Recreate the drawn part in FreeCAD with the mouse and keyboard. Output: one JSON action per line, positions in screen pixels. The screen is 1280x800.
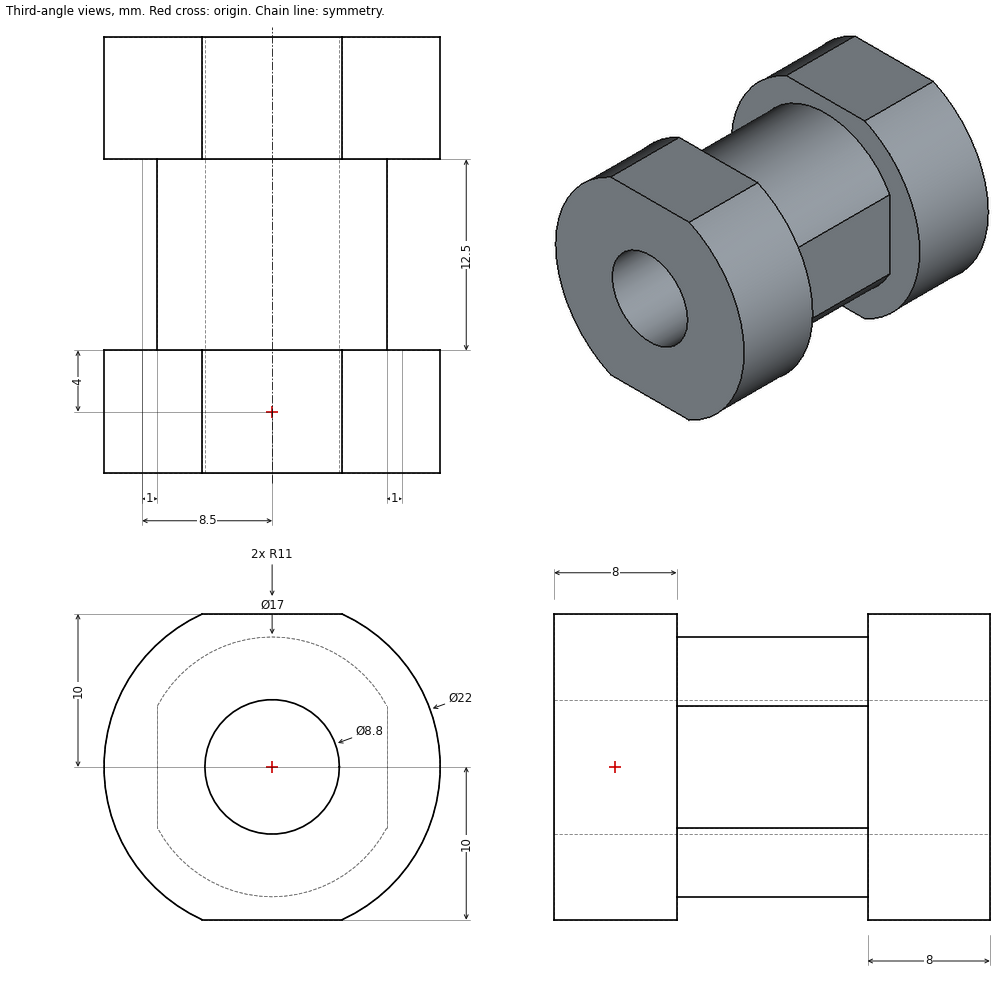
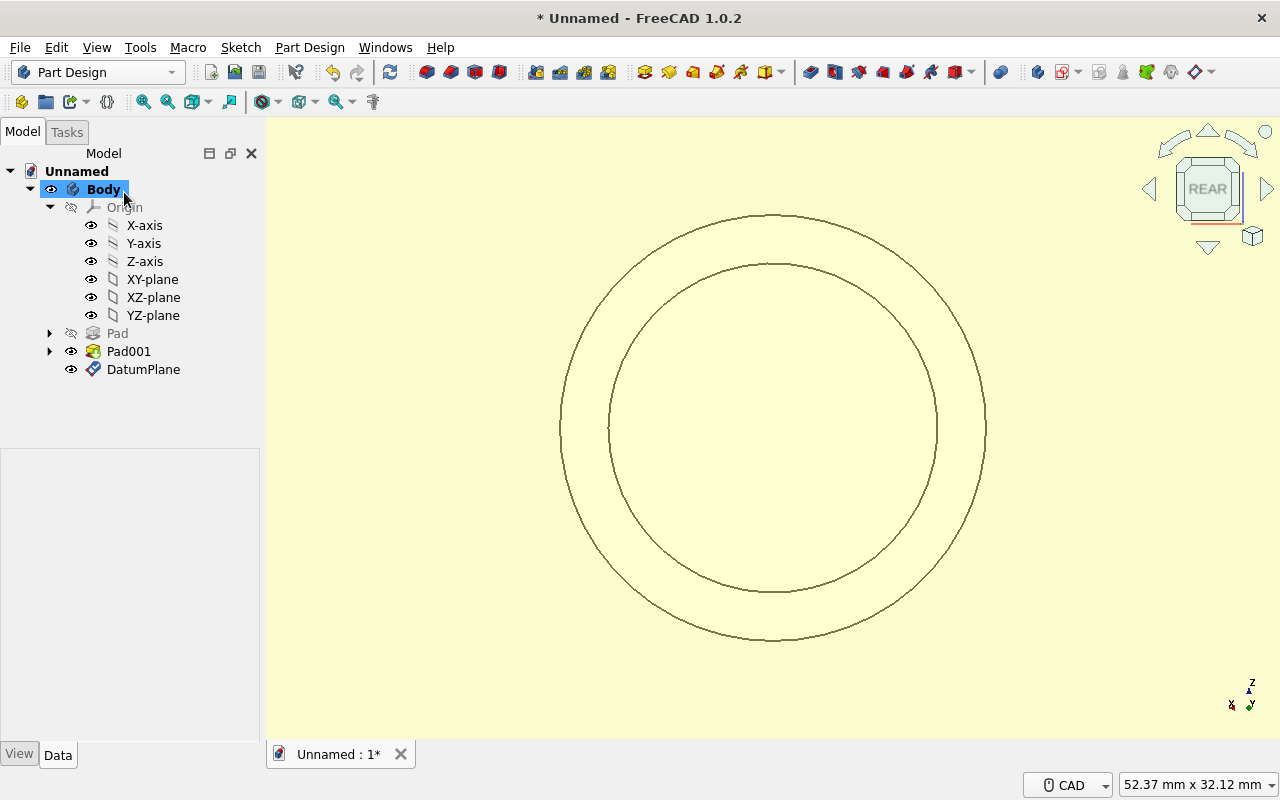
{"action": "left_click", "coordinate": [116, 369]}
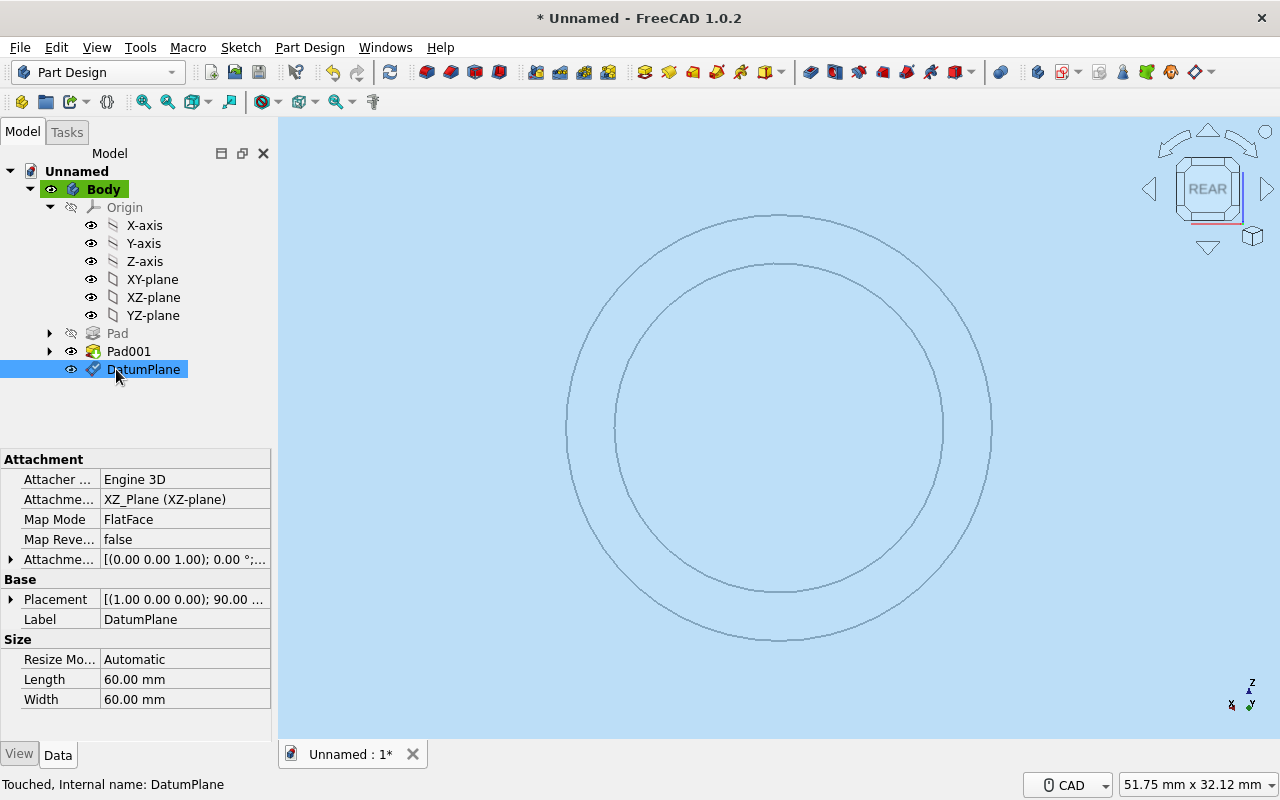
{"action": "left_click", "coordinate": [1062, 72]}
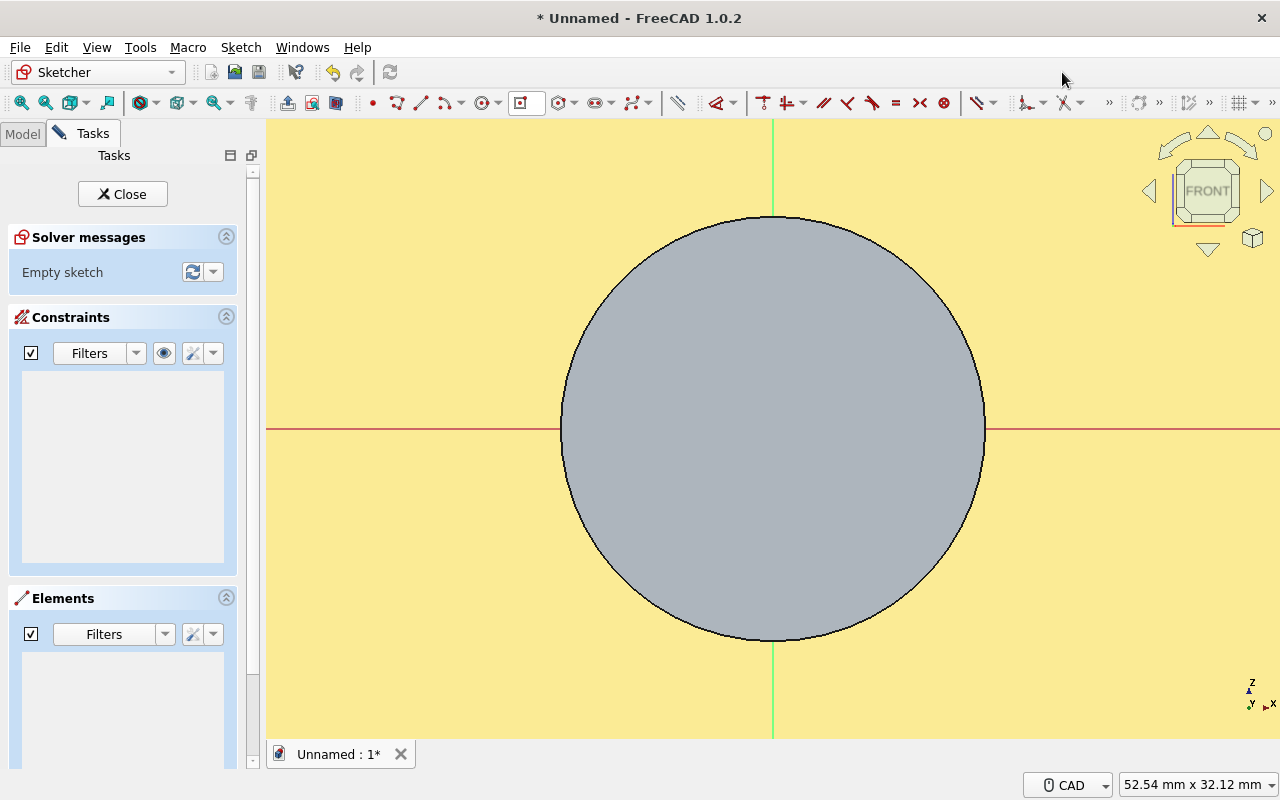
{"action": "key", "text": "q s"}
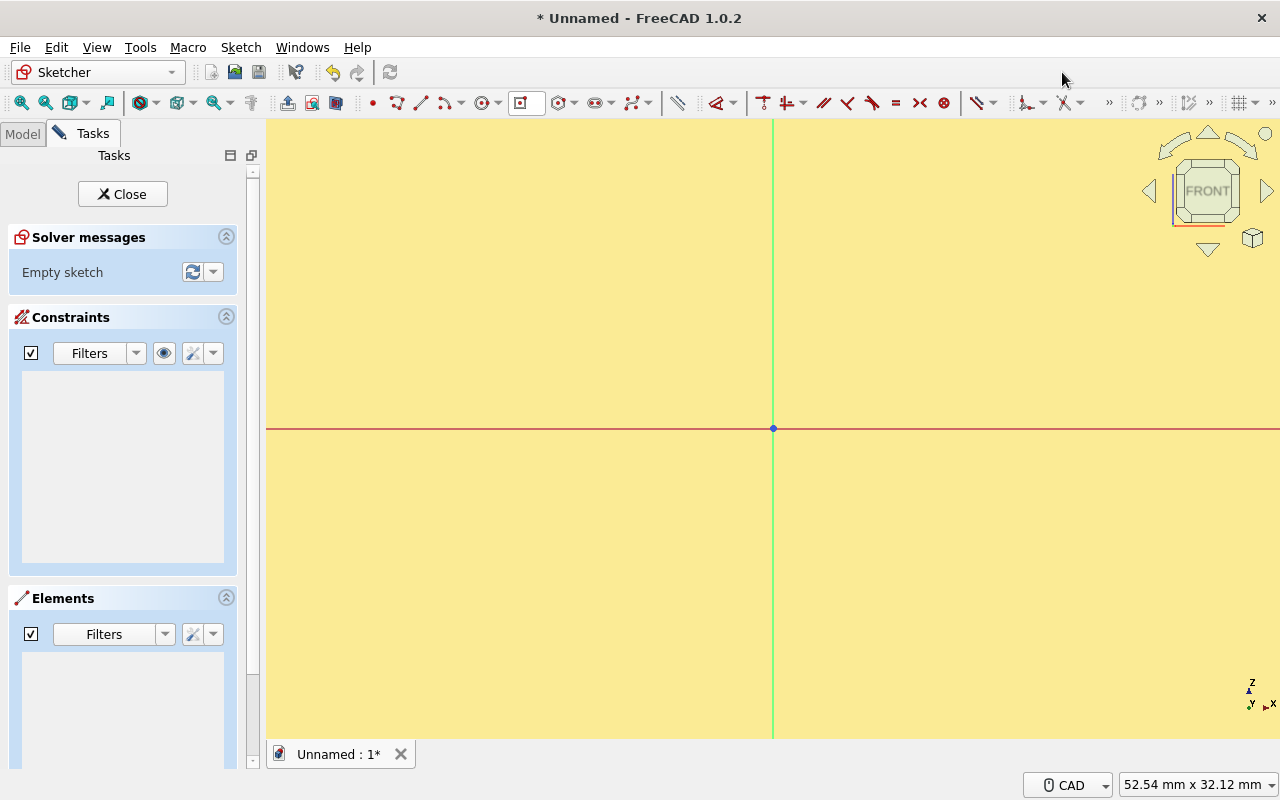
{"action": "left_click", "coordinate": [482, 104]}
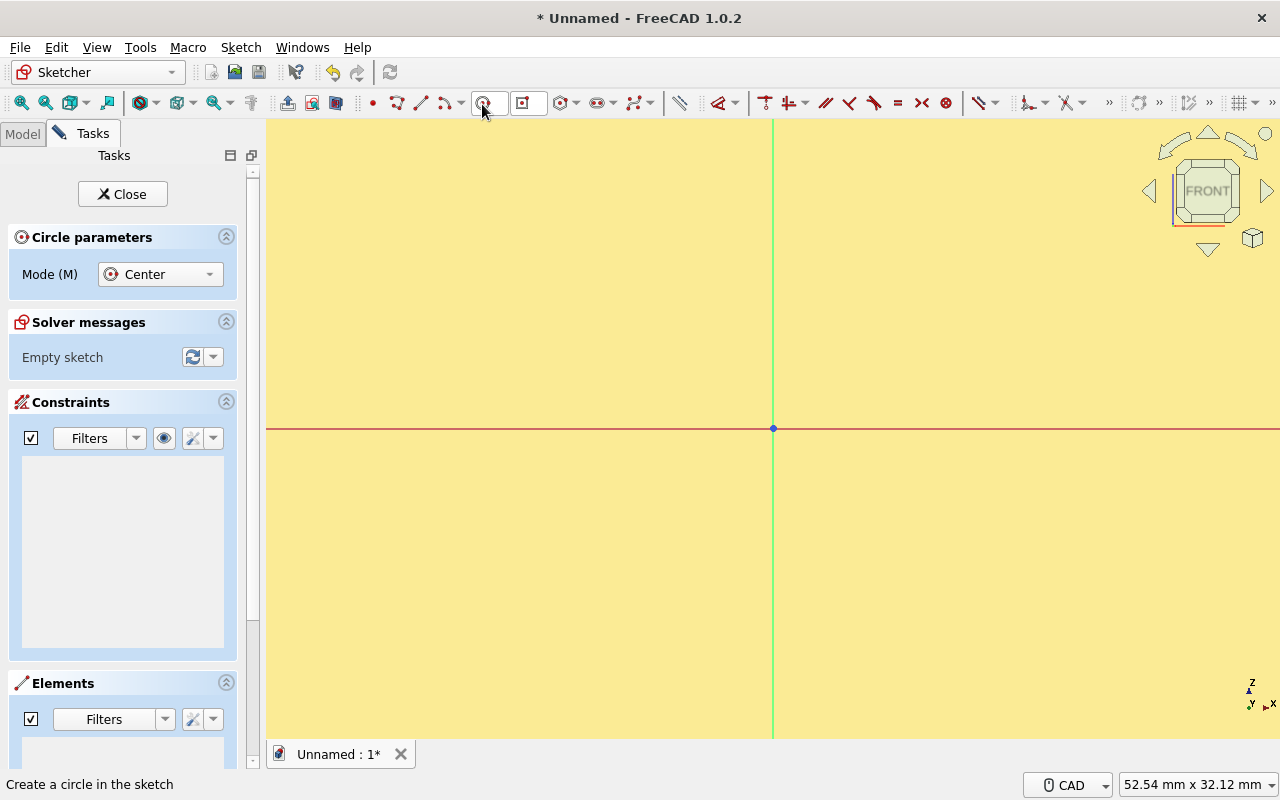
{"action": "left_click", "coordinate": [773, 429]}
{"action": "mouse_move", "coordinate": [923, 279]}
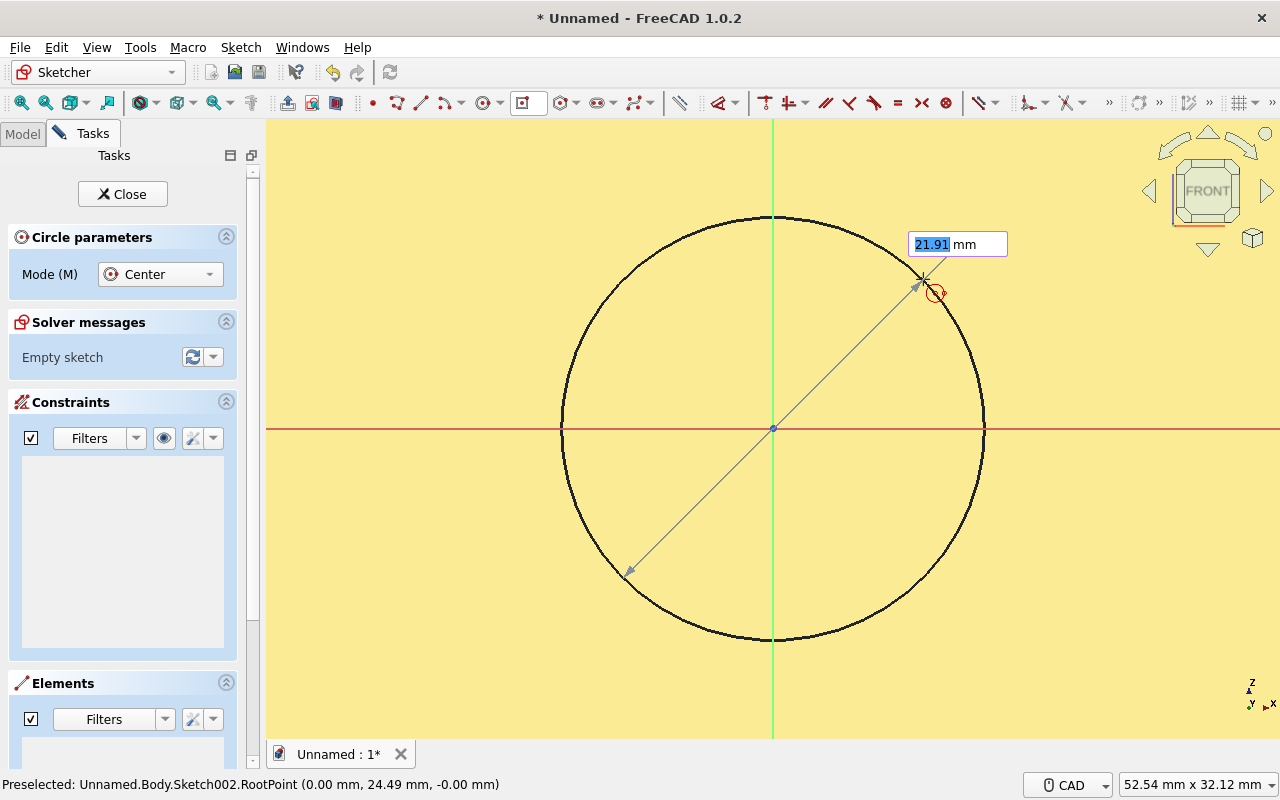
{"action": "type", "text": "22"}
{"action": "key", "text": "Return"}
{"action": "key", "text": "Escape"}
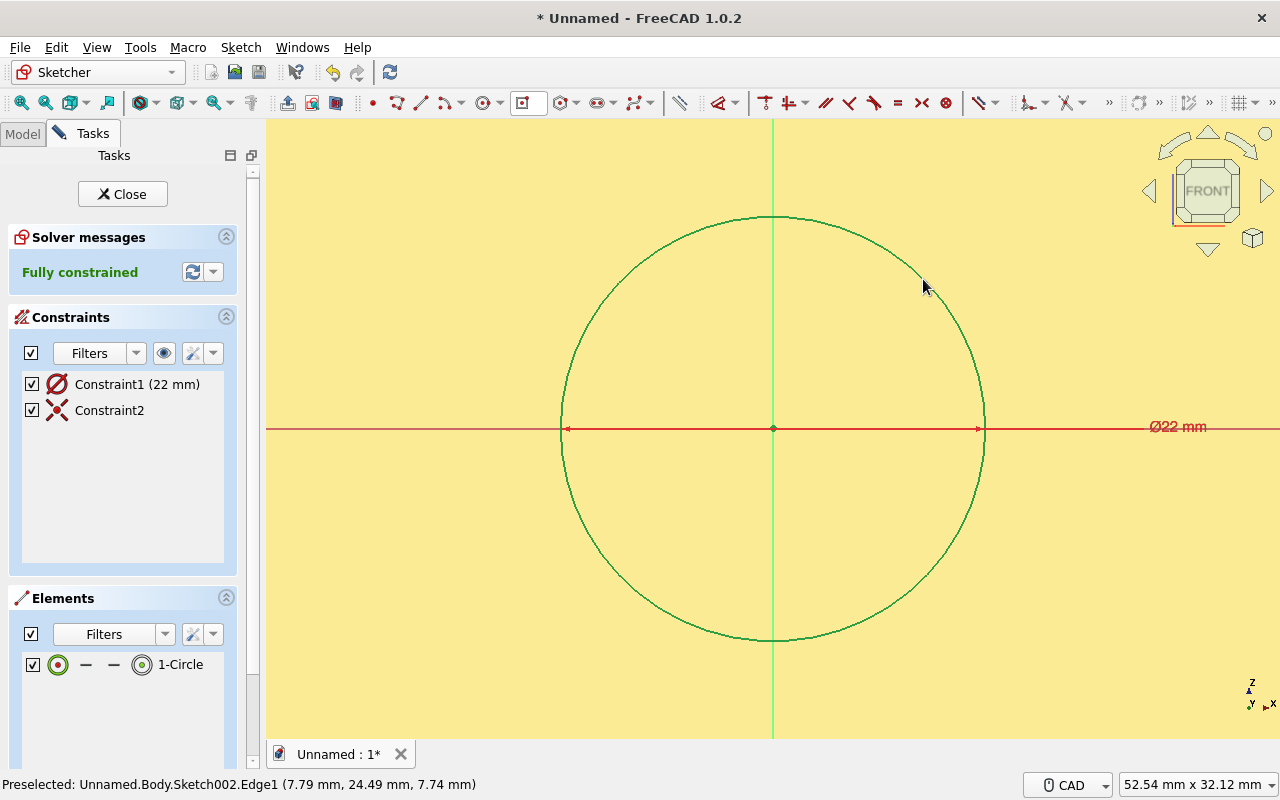
{"action": "left_click", "coordinate": [123, 194]}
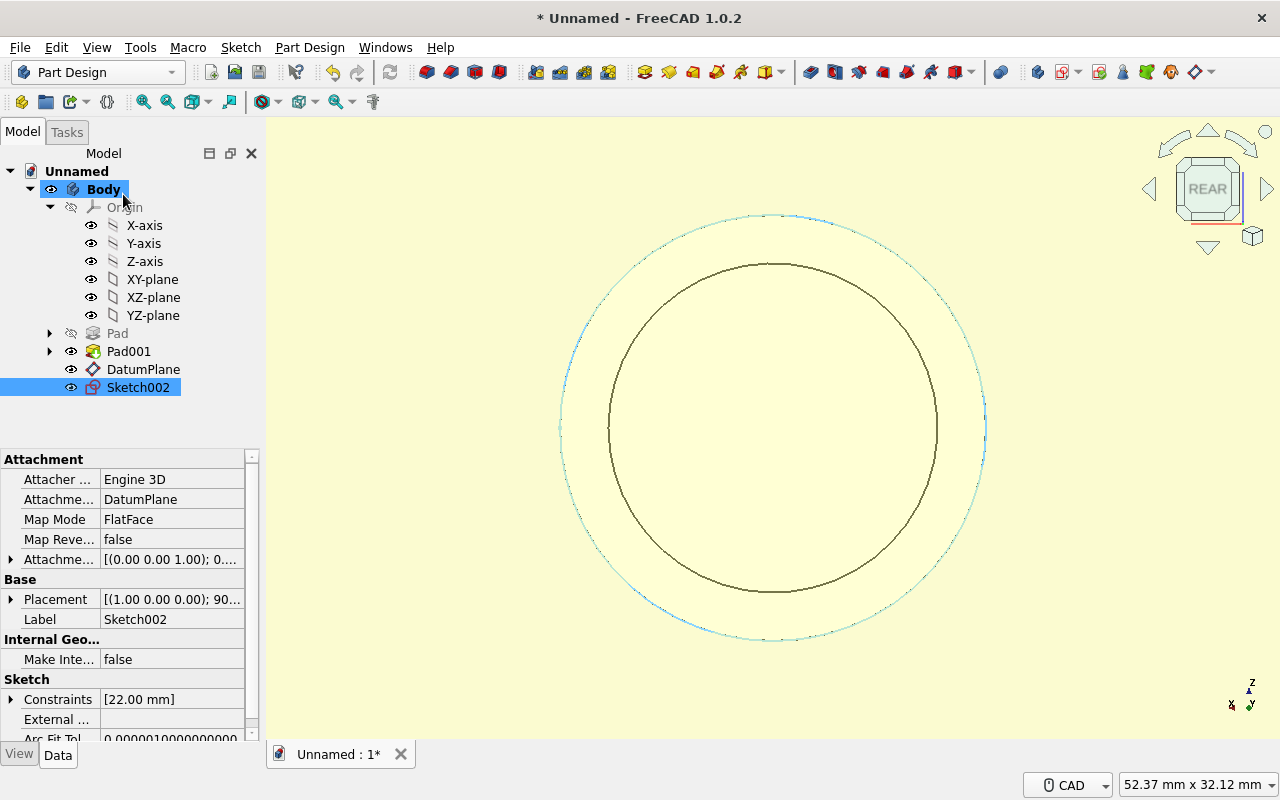
{"action": "left_click", "coordinate": [646, 72]}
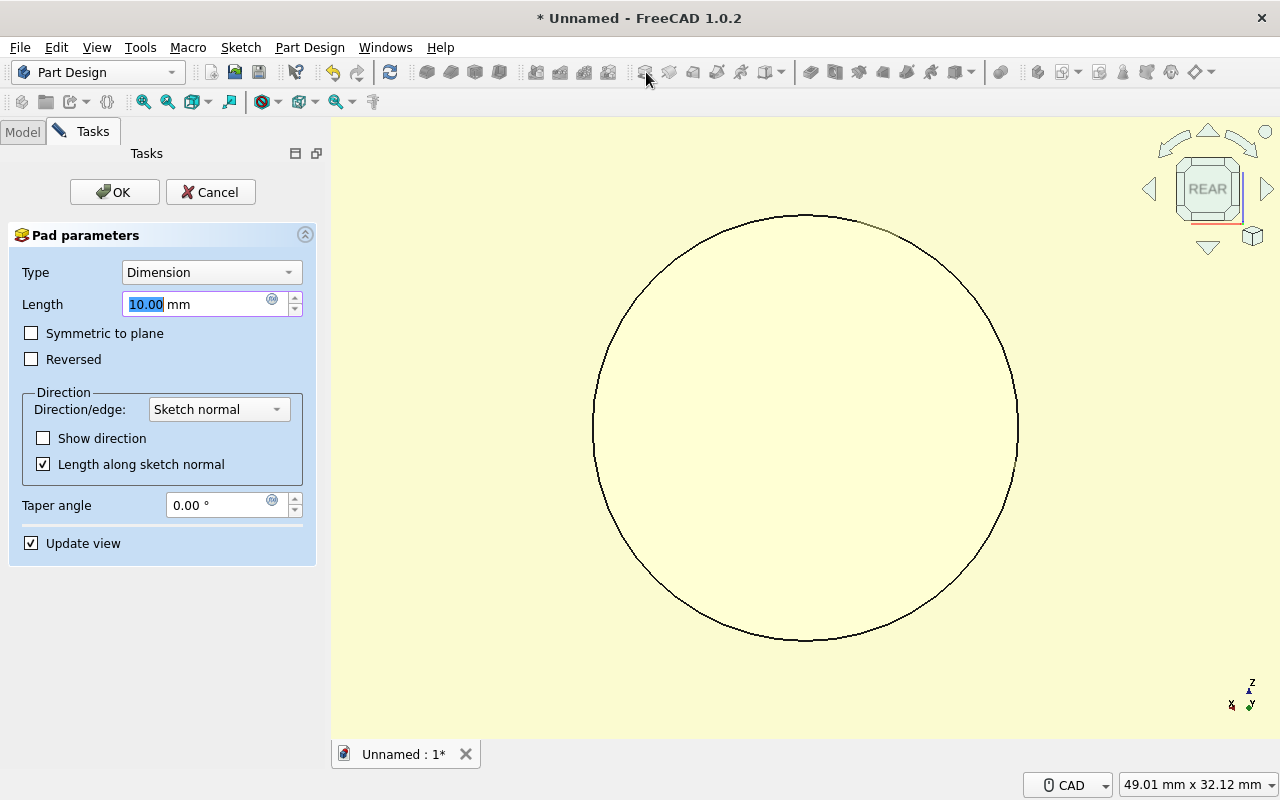
{"action": "type", "text": "8"}
{"action": "key", "text": "Tab"}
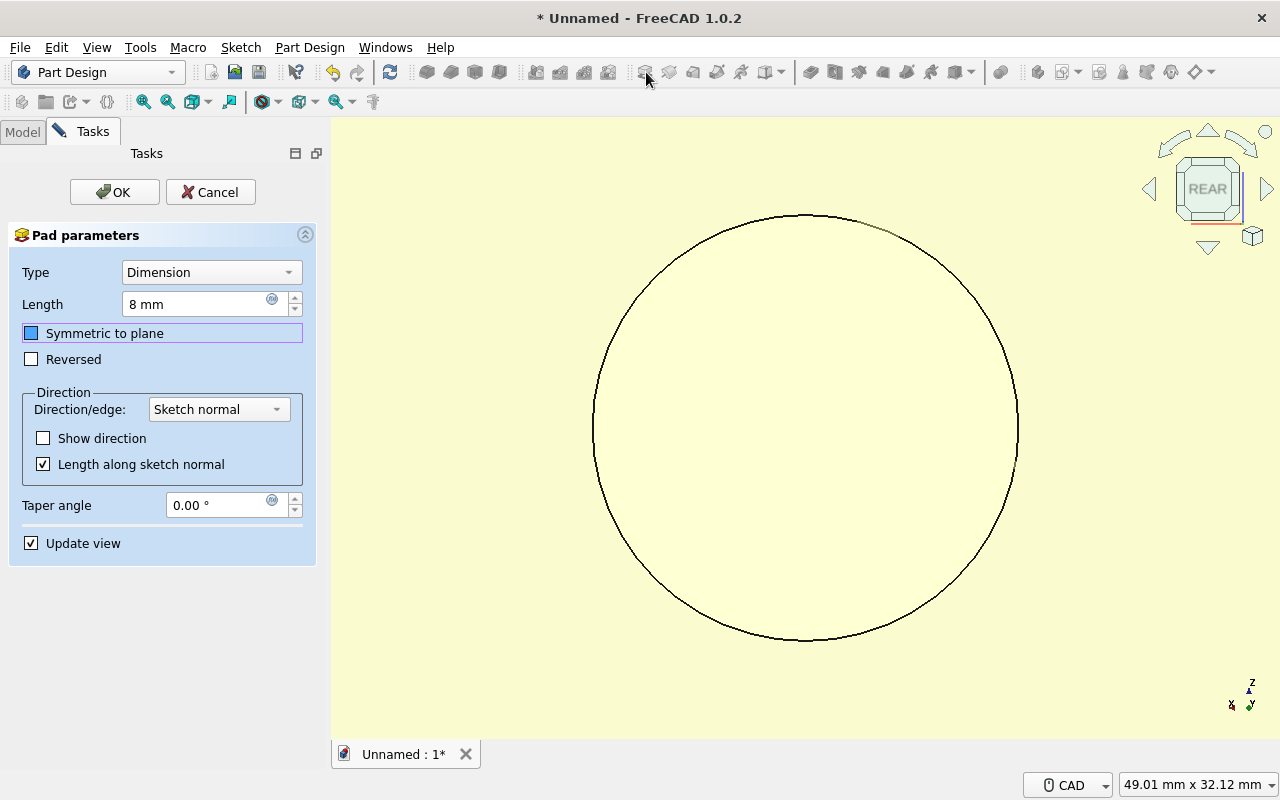
{"action": "left_click", "coordinate": [115, 192]}